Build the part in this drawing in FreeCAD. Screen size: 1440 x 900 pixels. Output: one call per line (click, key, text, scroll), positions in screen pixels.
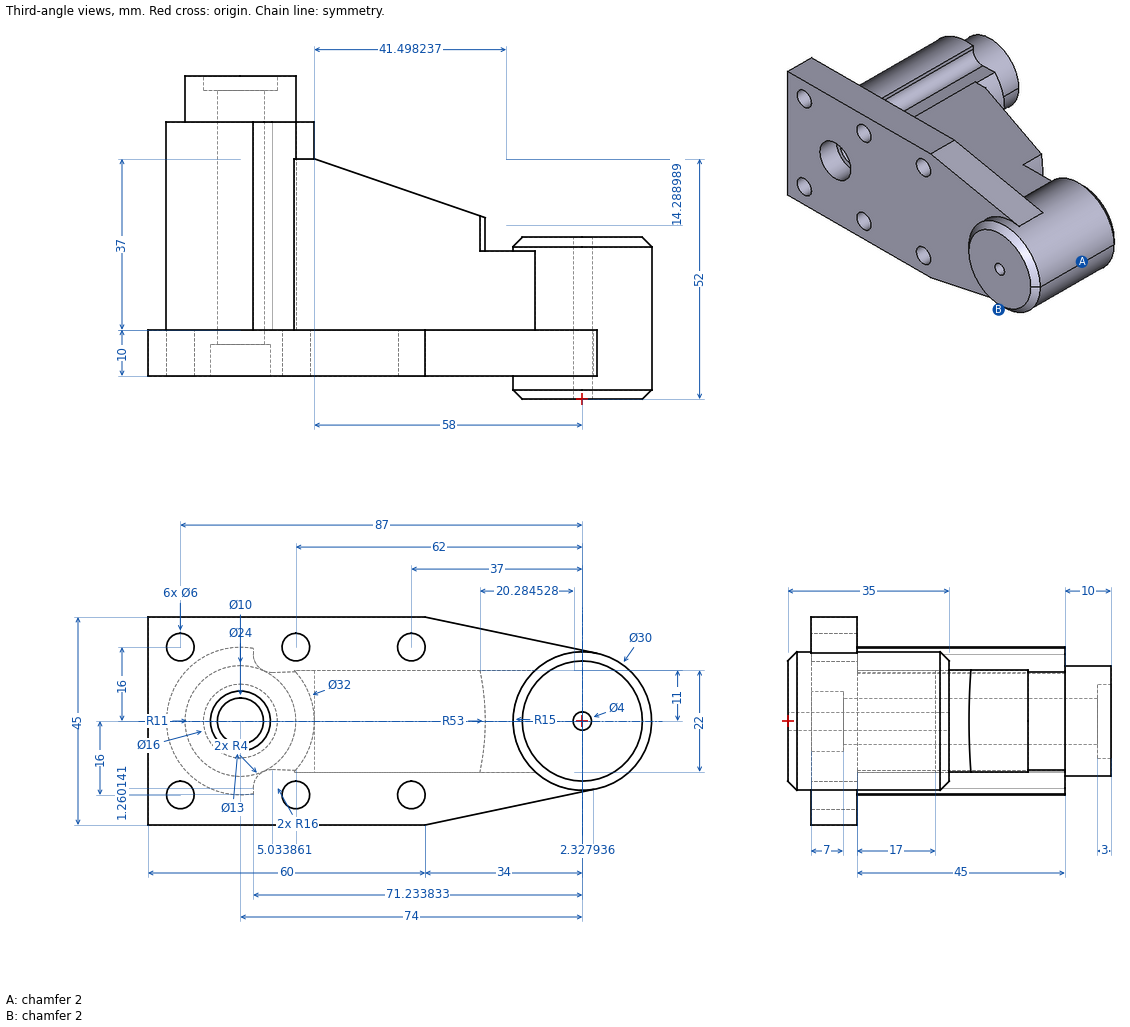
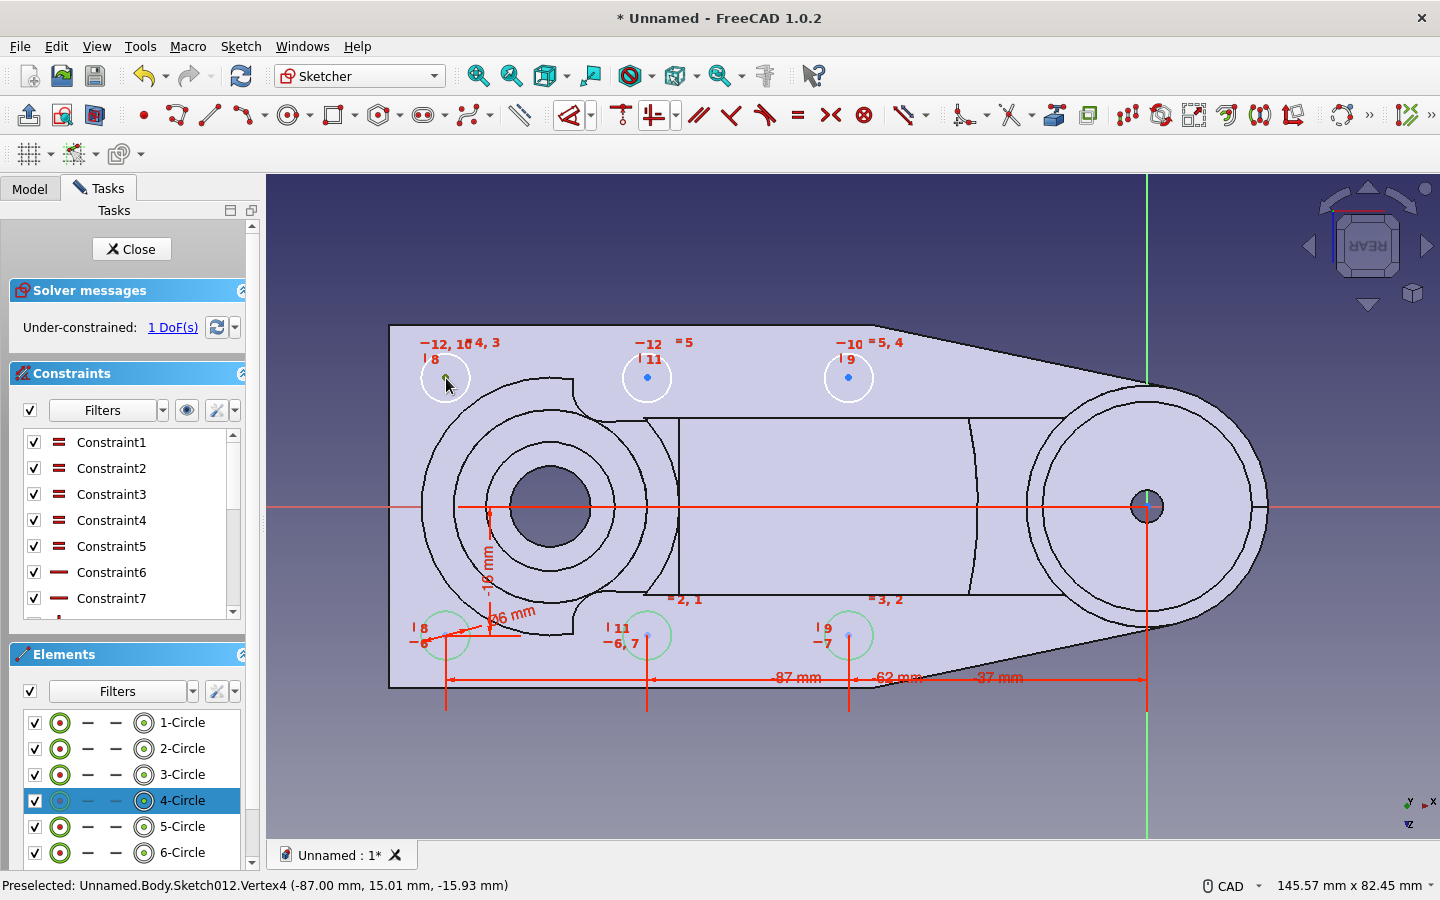
key(i)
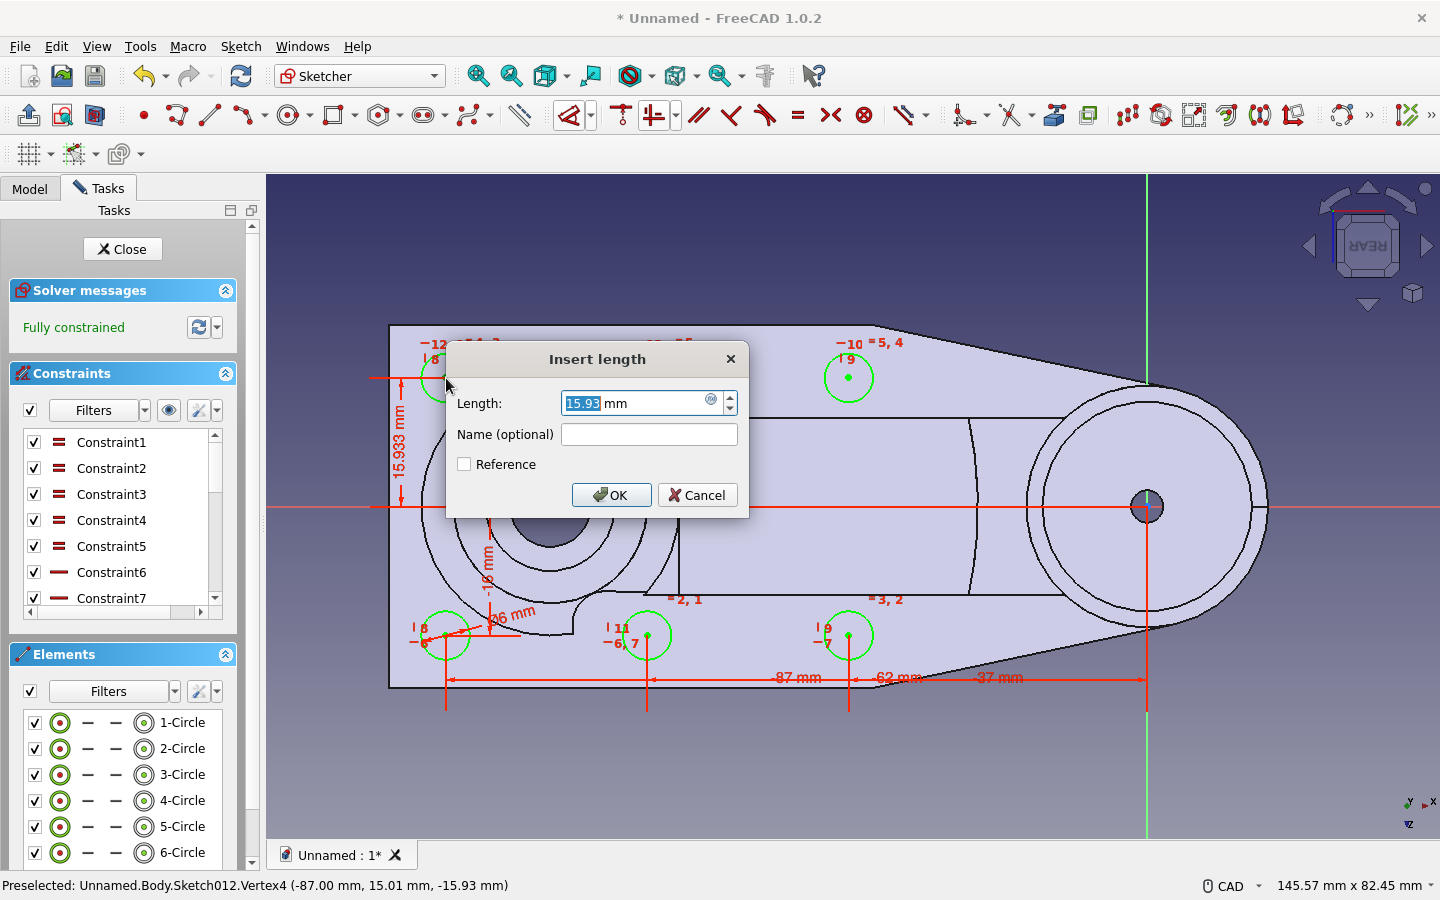
text(16)
key(Return)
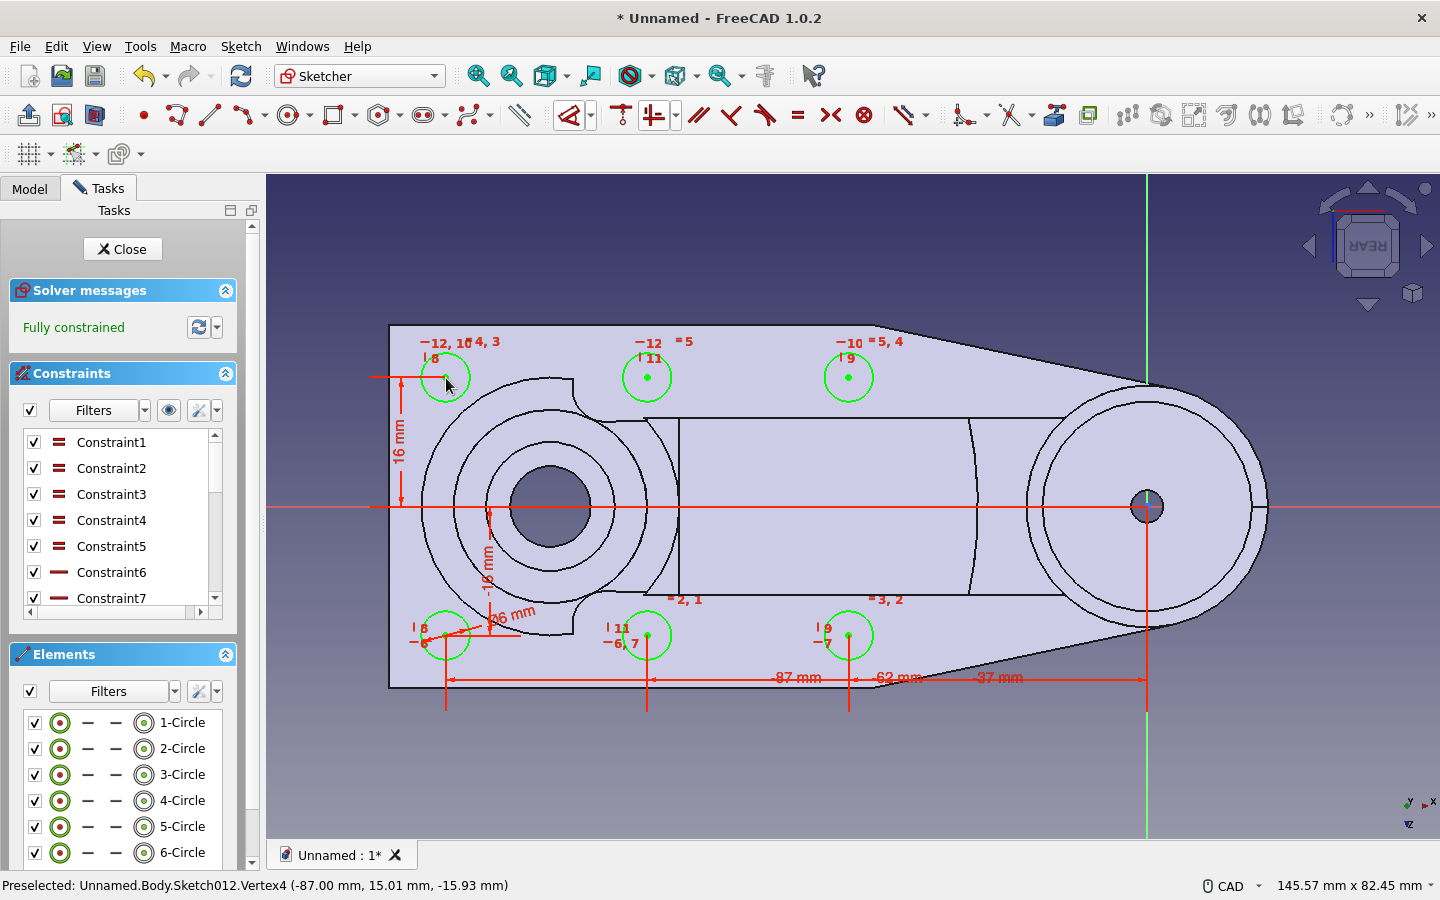
click(123, 249)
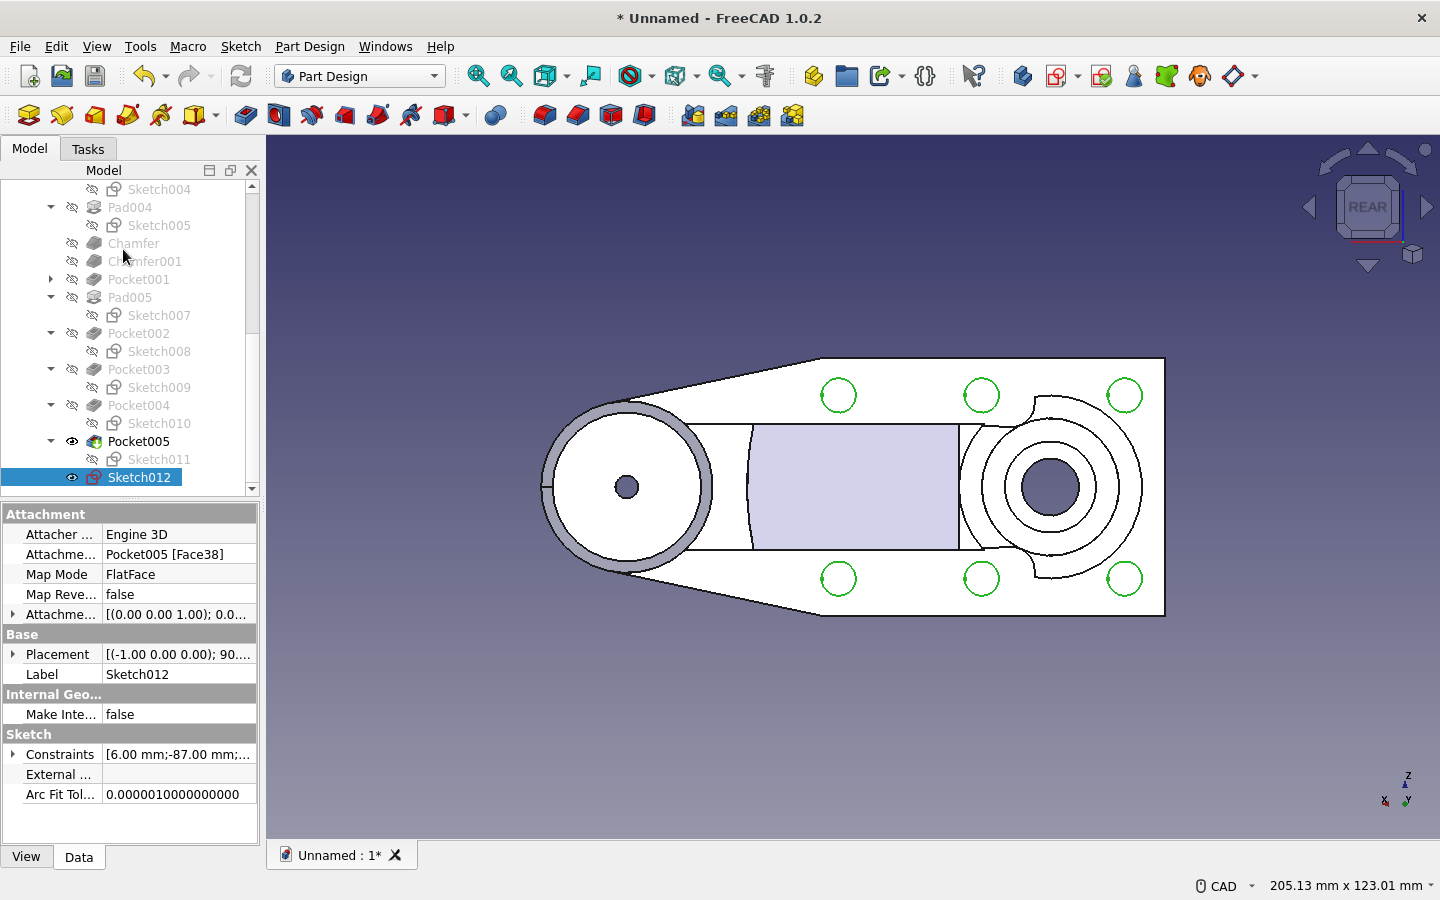
click(246, 116)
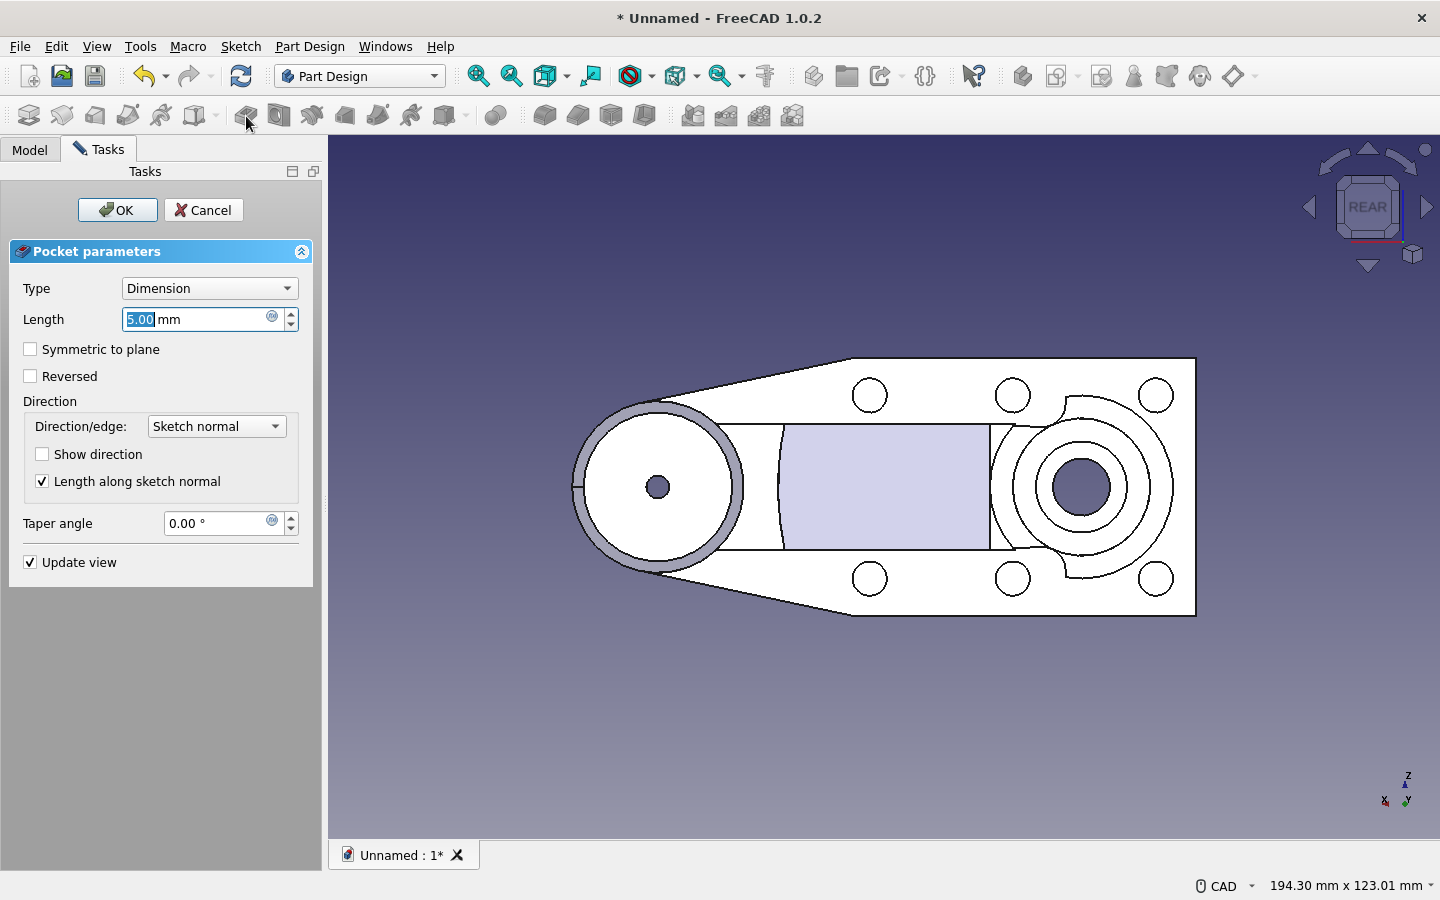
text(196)
key(Tab)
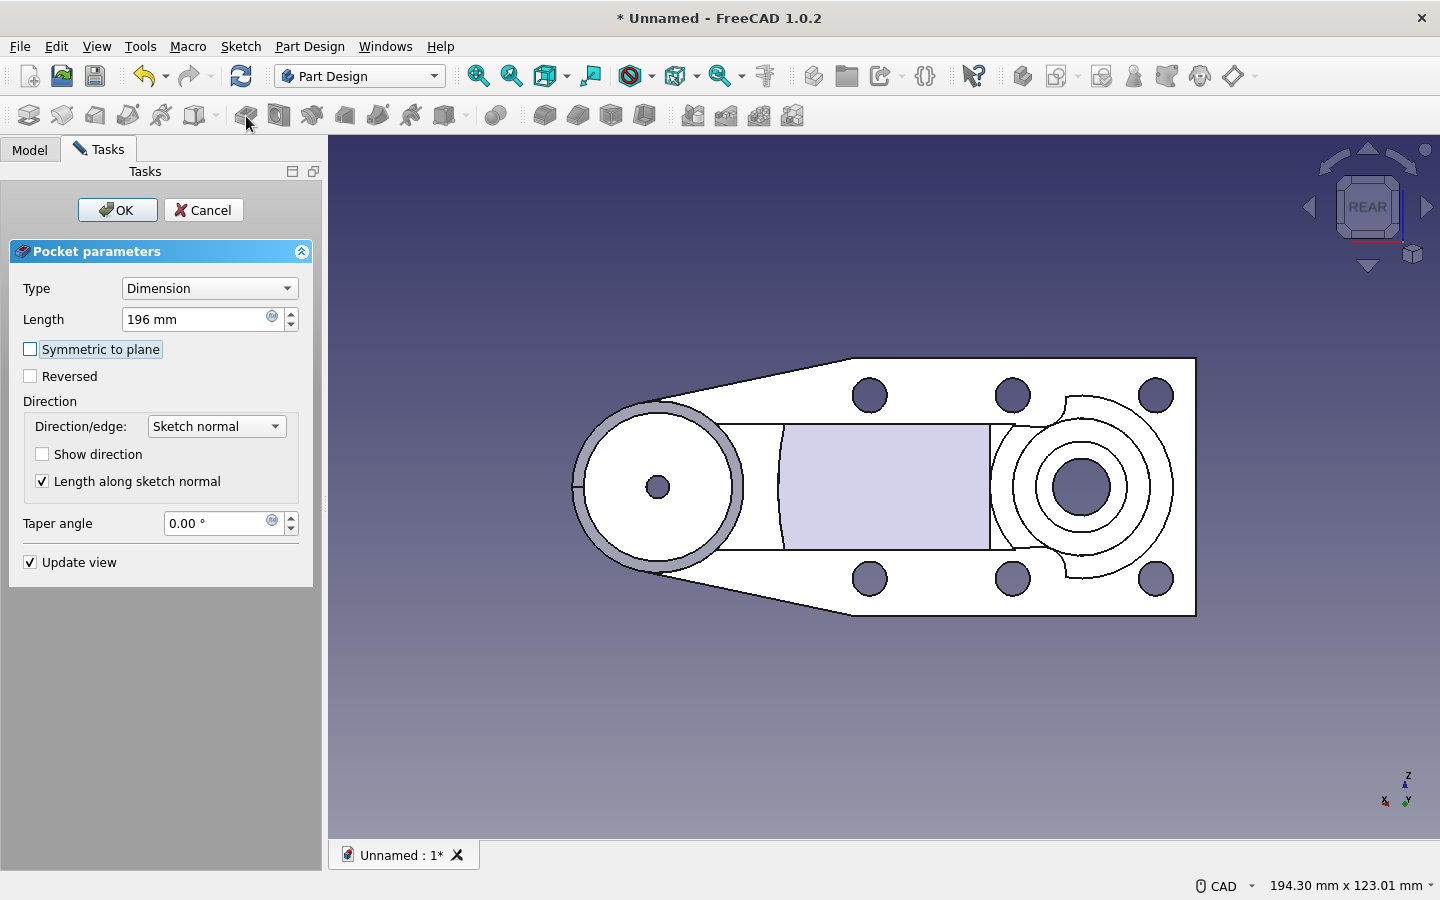
click(118, 210)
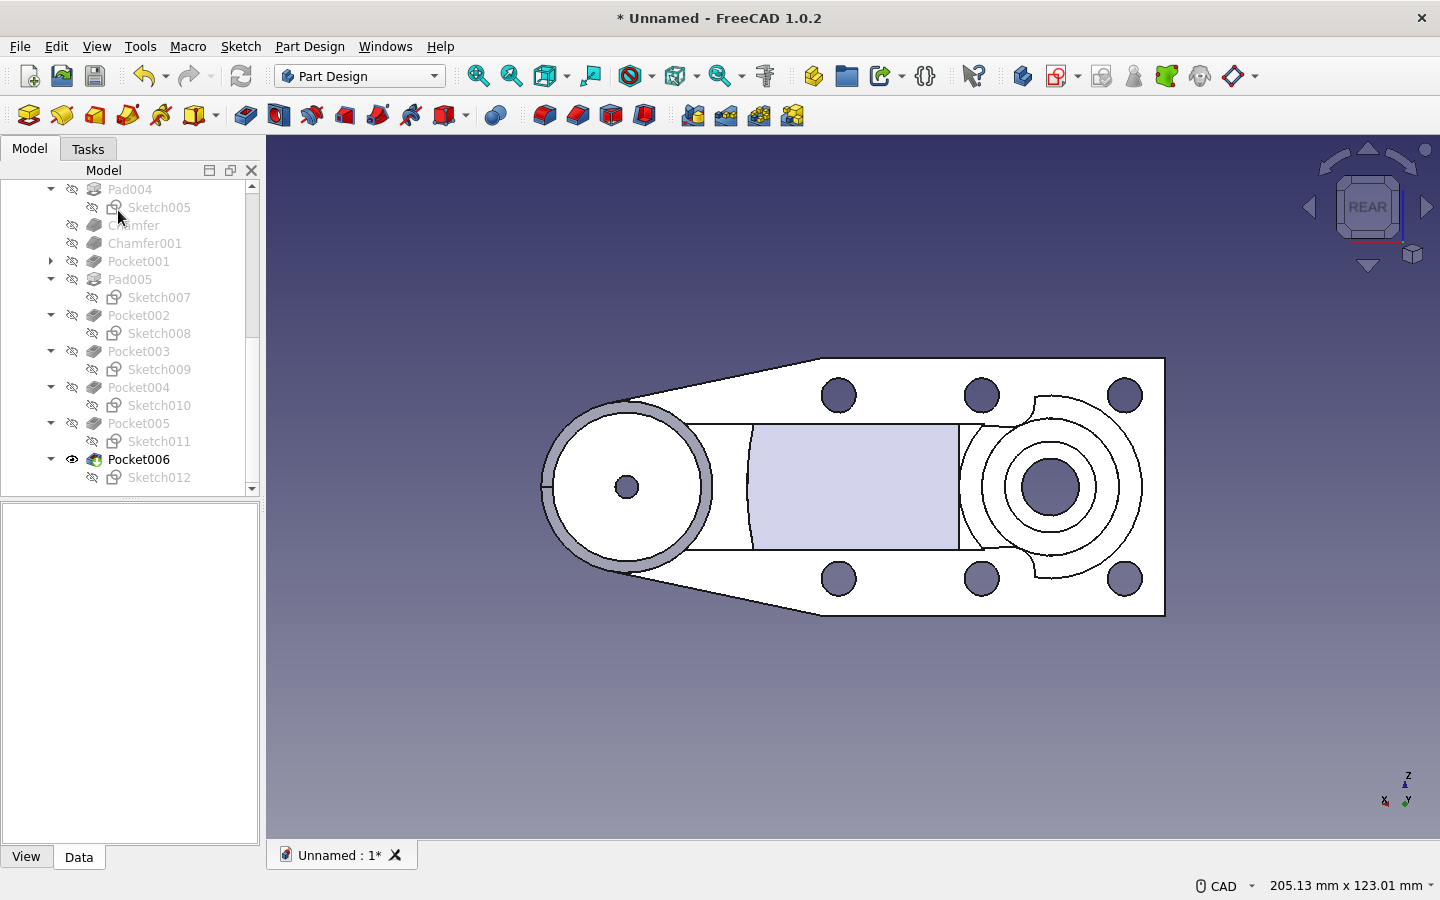
key(0)